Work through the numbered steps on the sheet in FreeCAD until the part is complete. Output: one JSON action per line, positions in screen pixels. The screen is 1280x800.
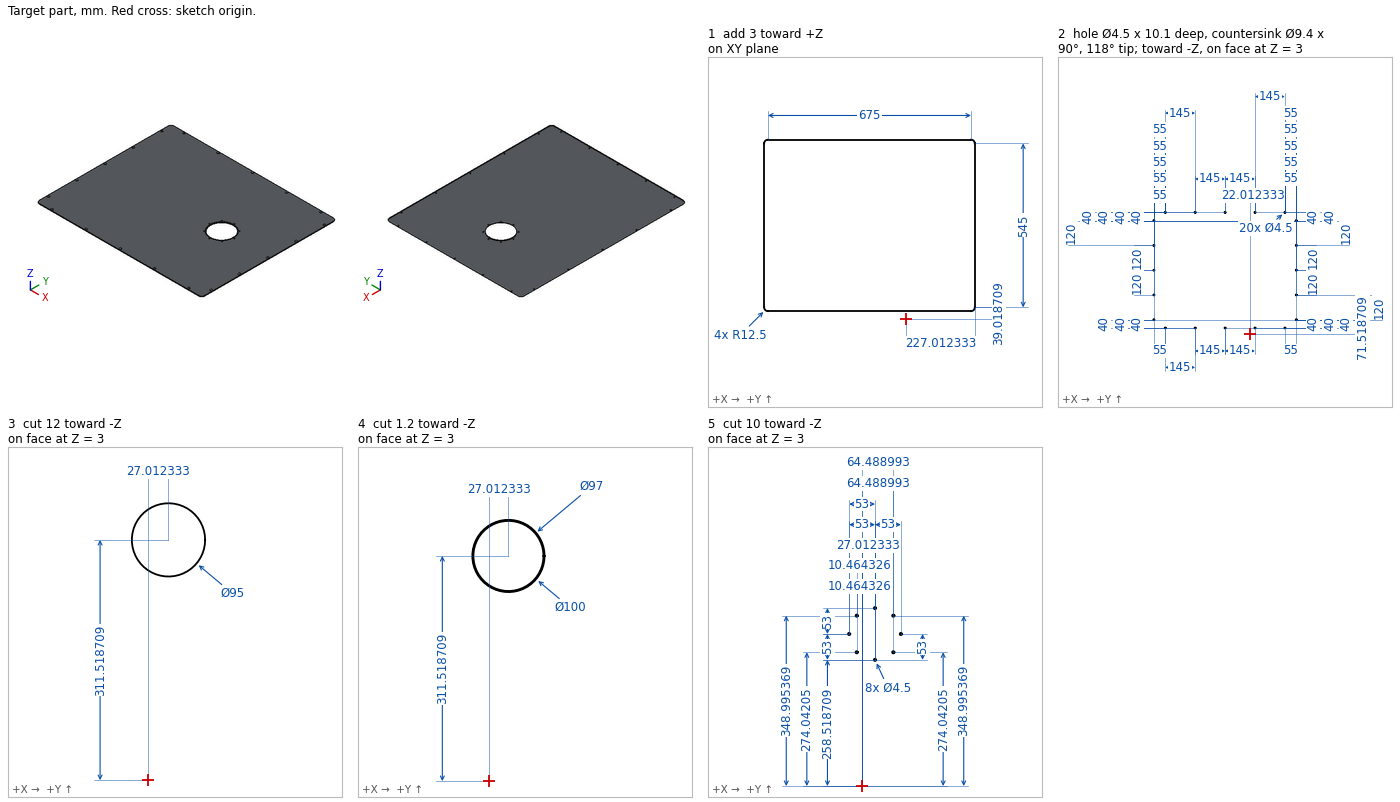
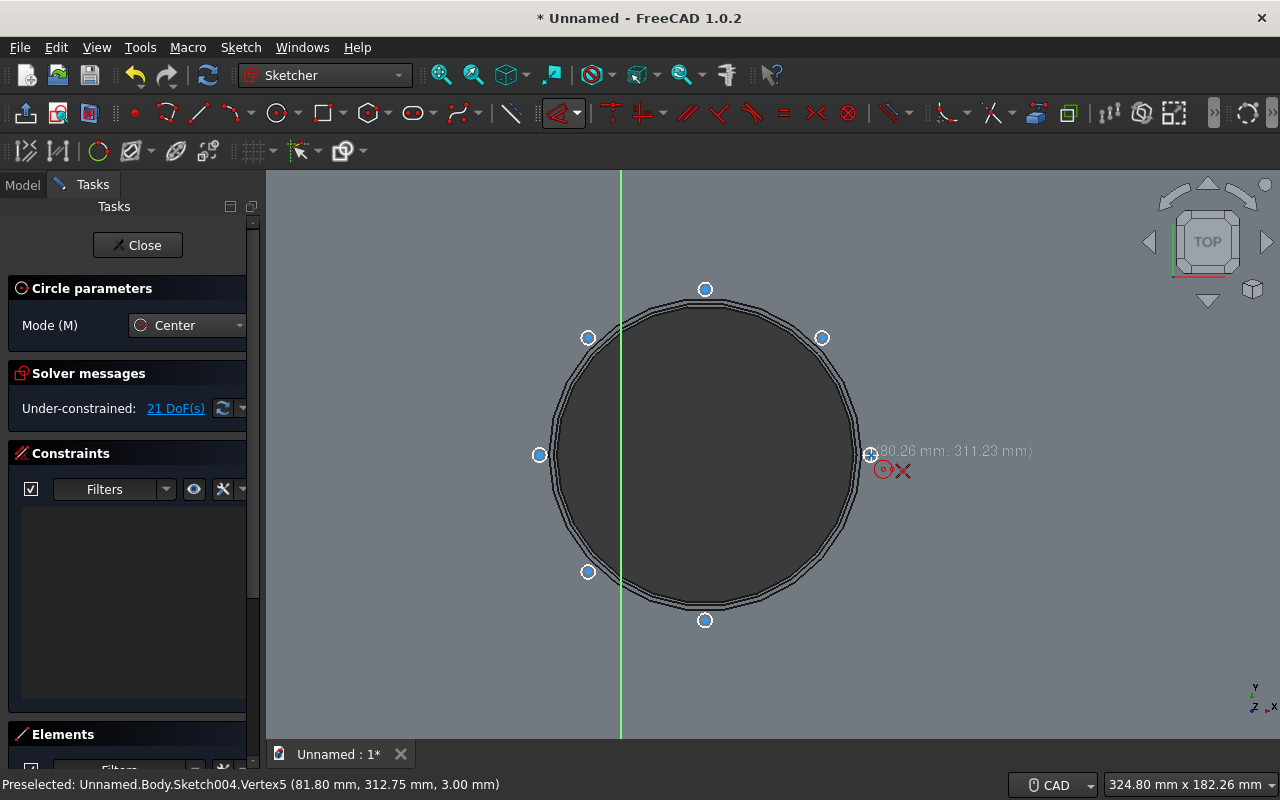
{"action": "scroll", "coordinate": [822, 572], "scroll_direction": "up", "scroll_amount": 6}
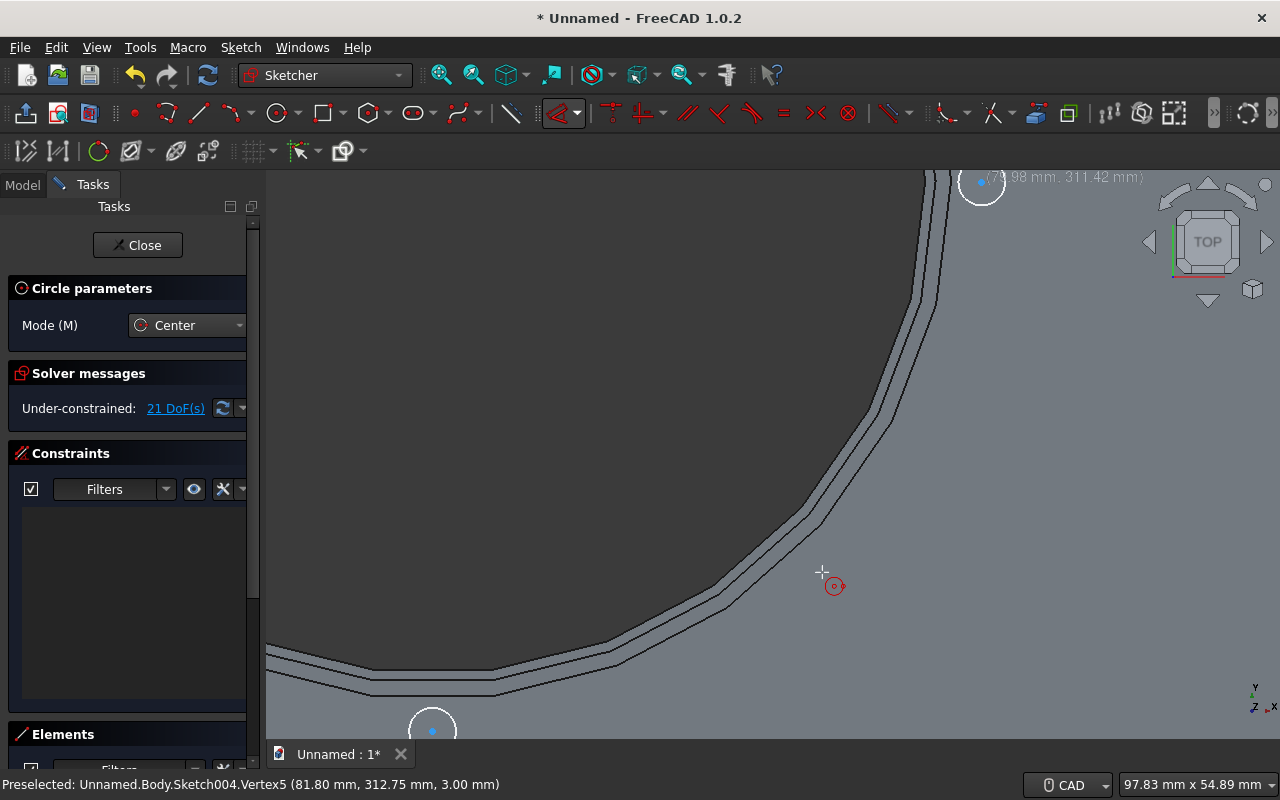
{"action": "left_click", "coordinate": [821, 570]}
{"action": "left_click", "coordinate": [838, 553]}
{"action": "key", "text": "Escape"}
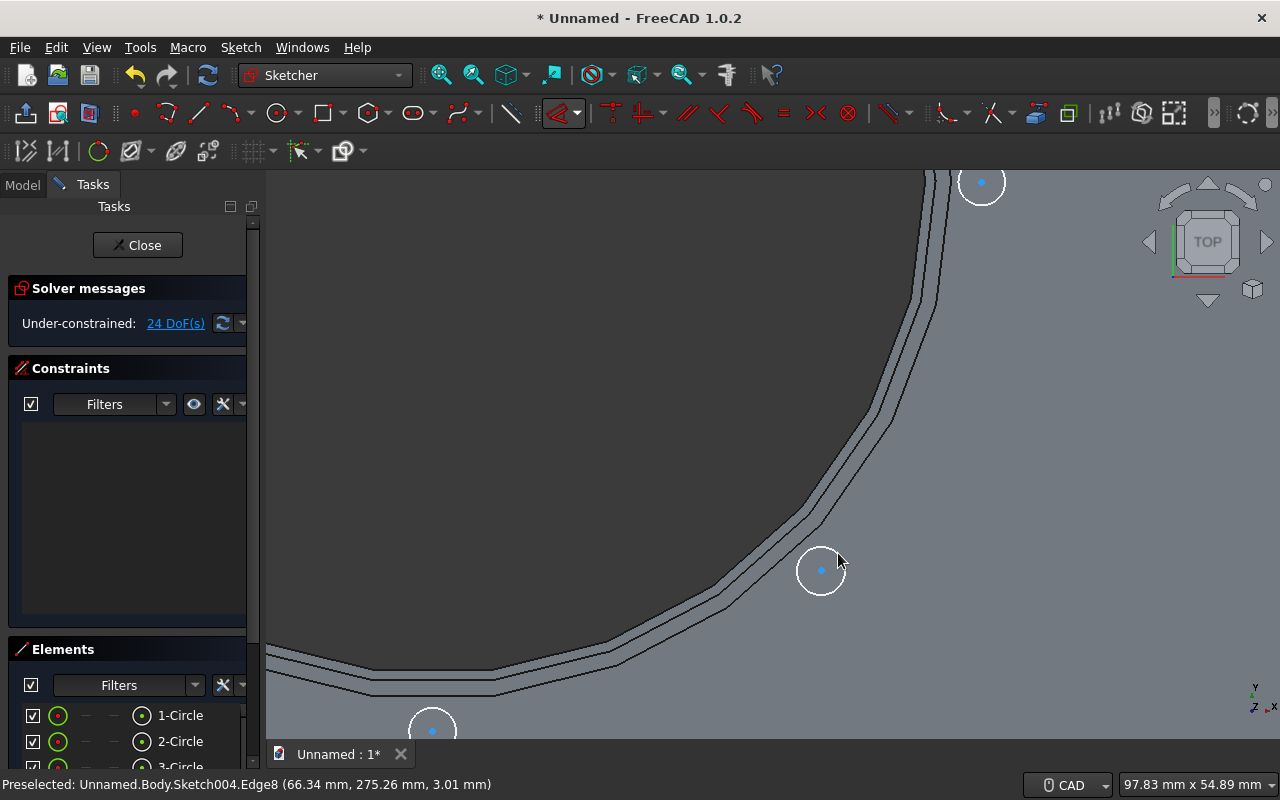
{"action": "left_click", "coordinate": [433, 708]}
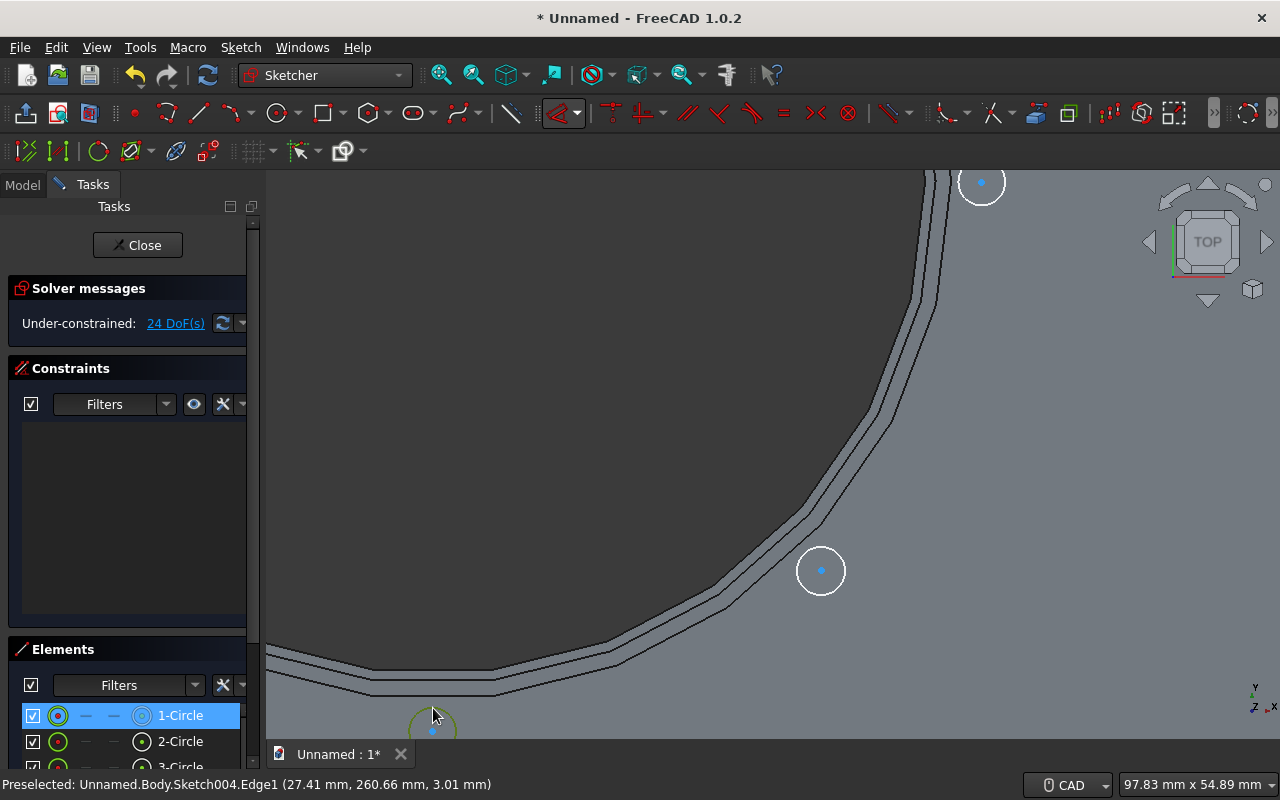
{"action": "scroll", "coordinate": [822, 572], "scroll_direction": "down", "scroll_amount": 6}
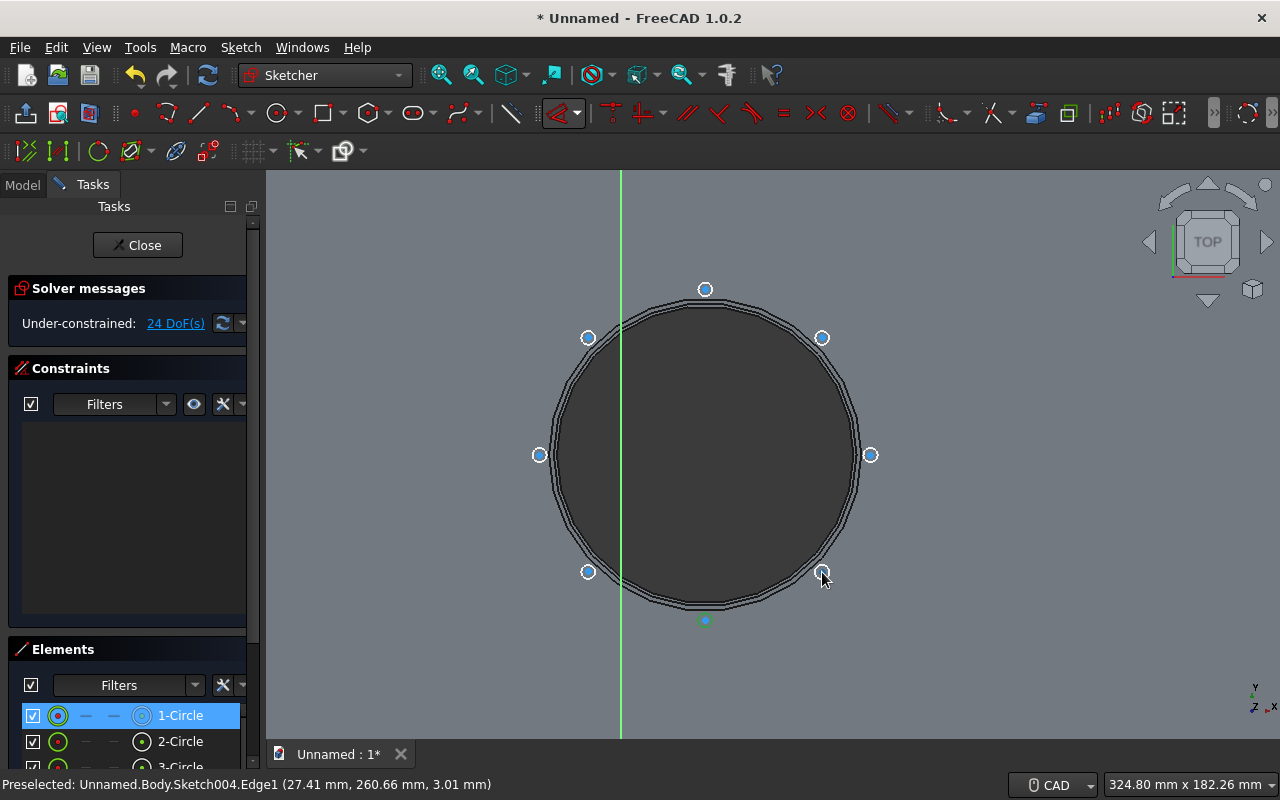
{"action": "scroll", "coordinate": [593, 567], "scroll_direction": "up", "scroll_amount": 4}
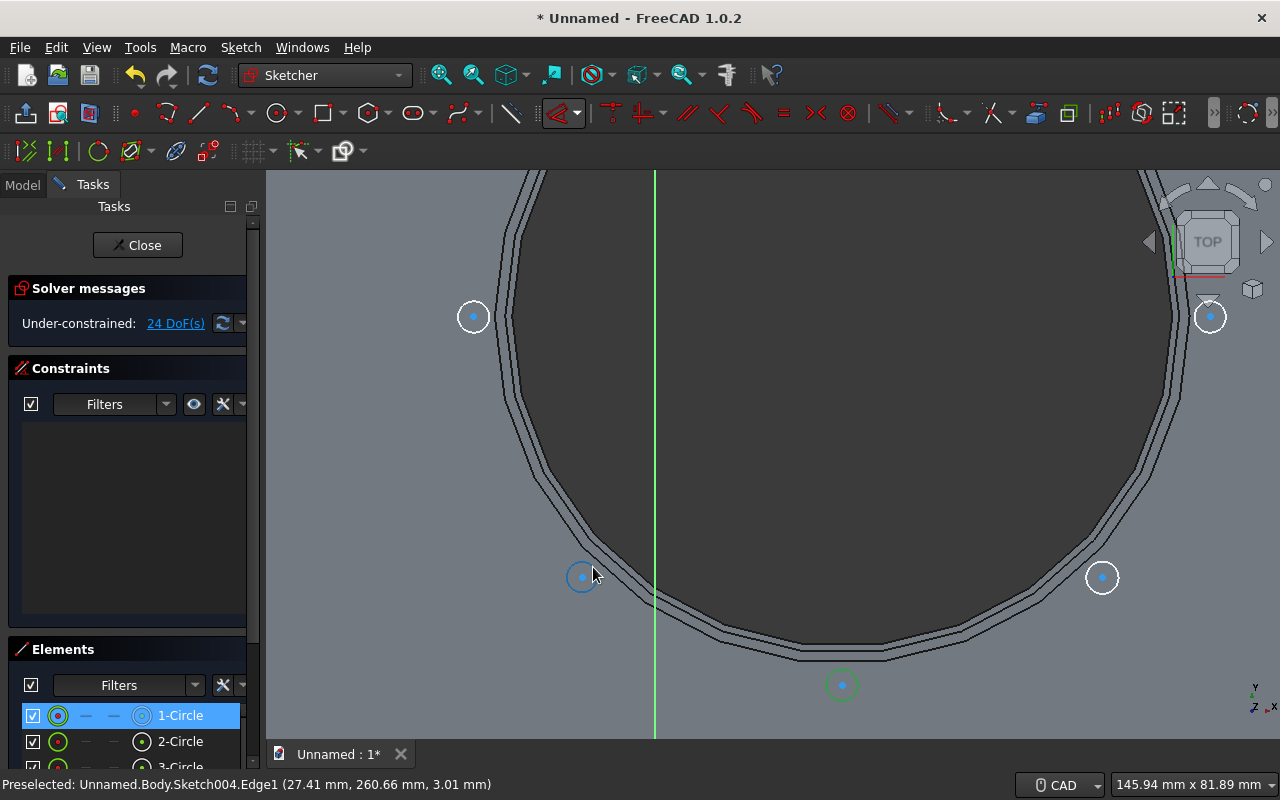
{"action": "left_click", "coordinate": [593, 566]}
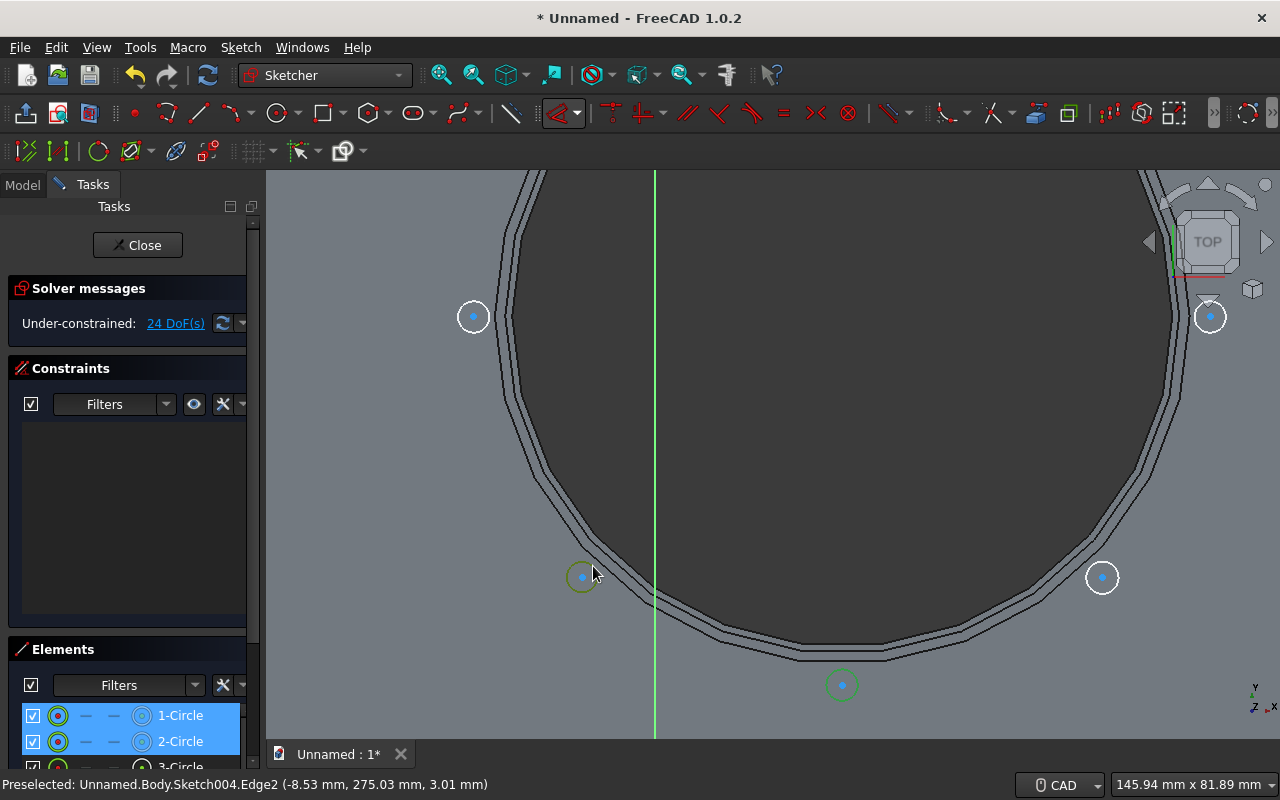
{"action": "left_click", "coordinate": [485, 306]}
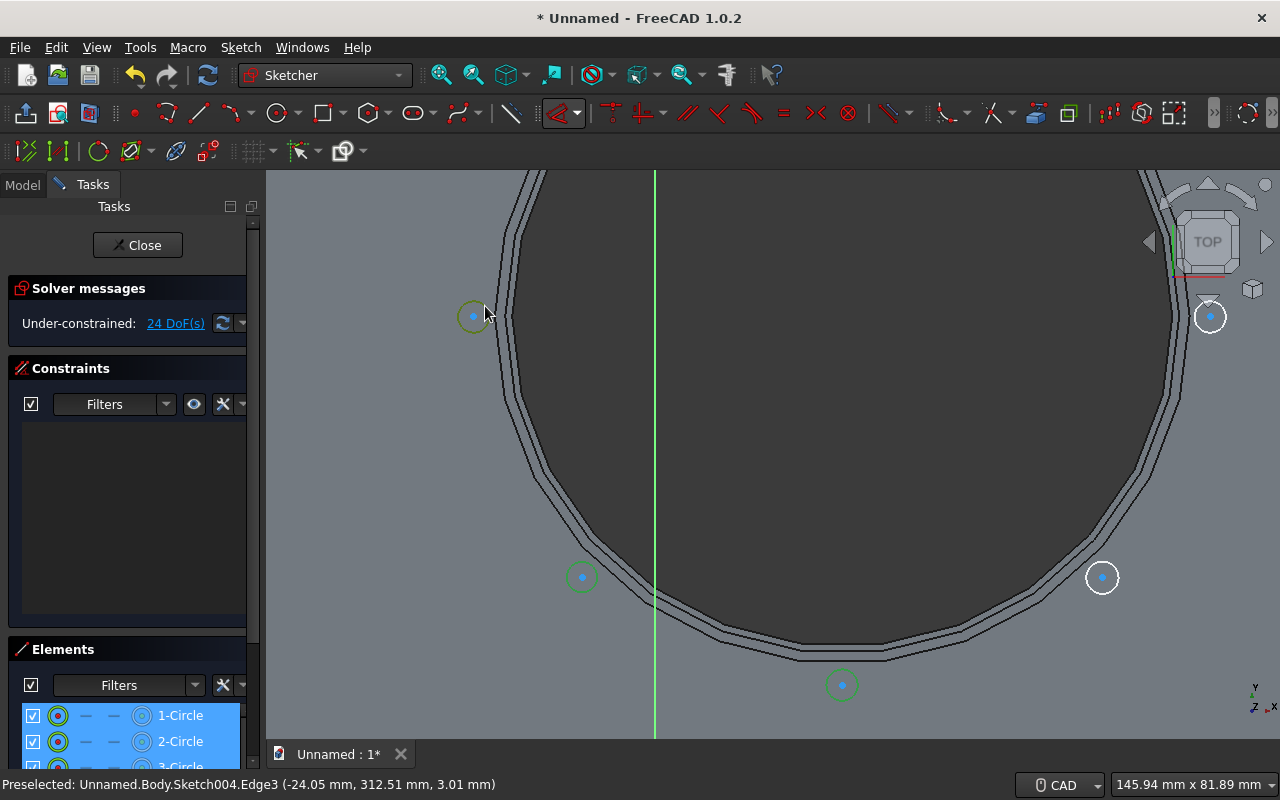
{"action": "scroll", "coordinate": [592, 567], "scroll_direction": "down", "scroll_amount": 4}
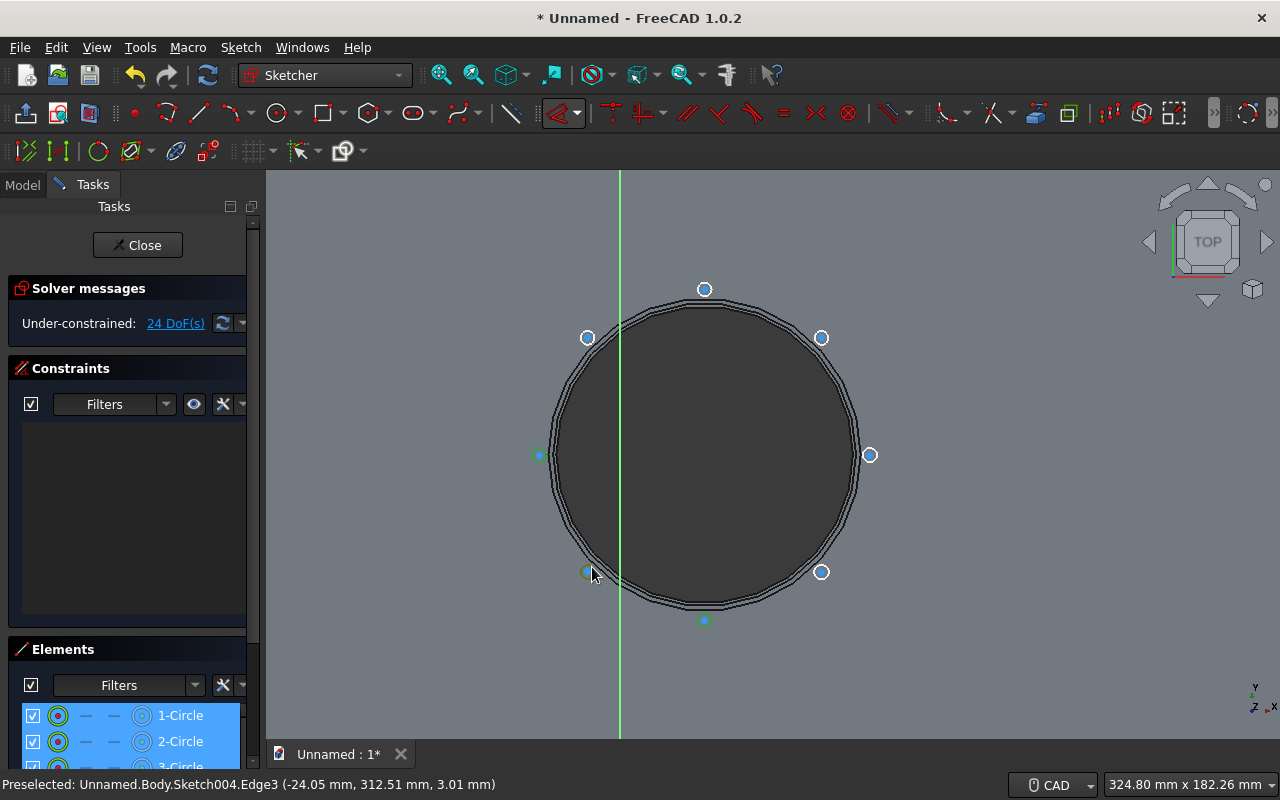
{"action": "scroll", "coordinate": [592, 333], "scroll_direction": "up", "scroll_amount": 4}